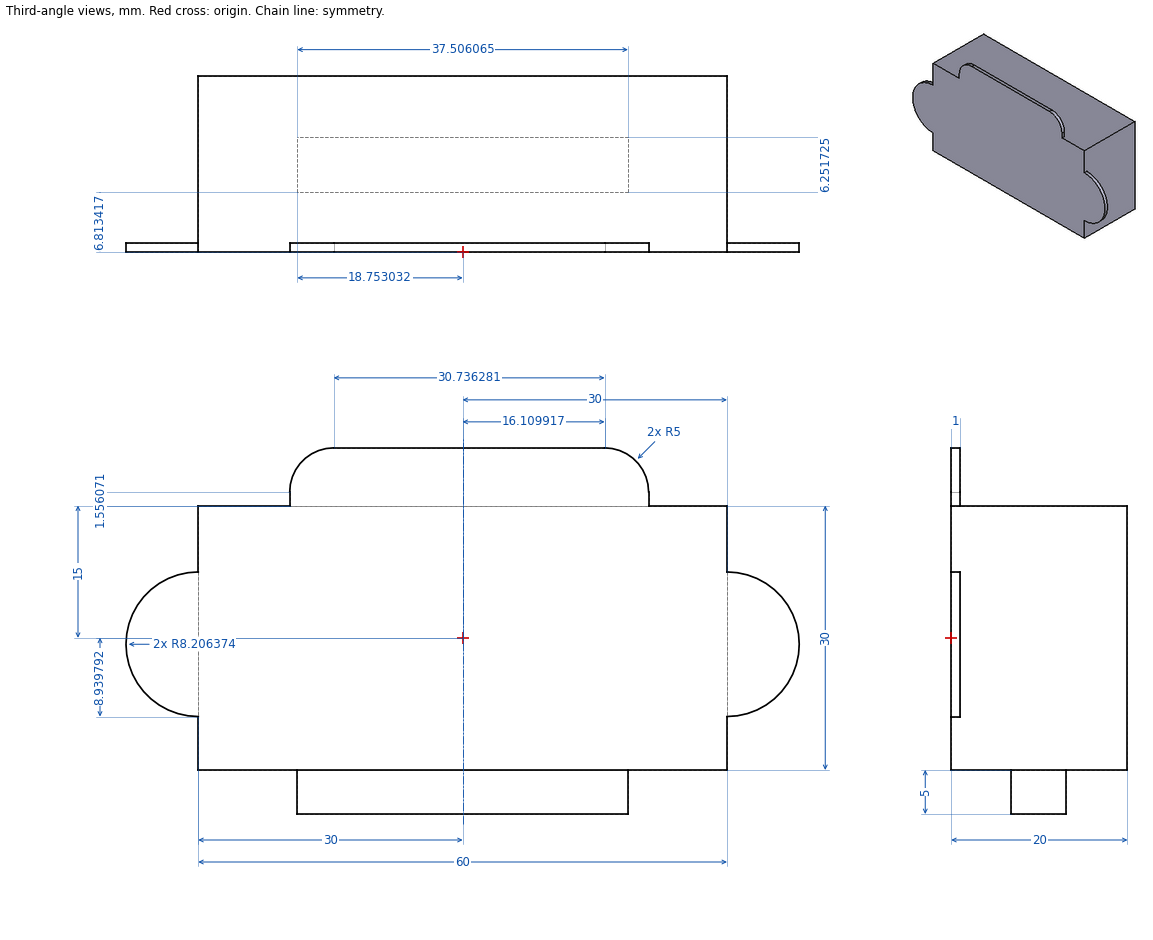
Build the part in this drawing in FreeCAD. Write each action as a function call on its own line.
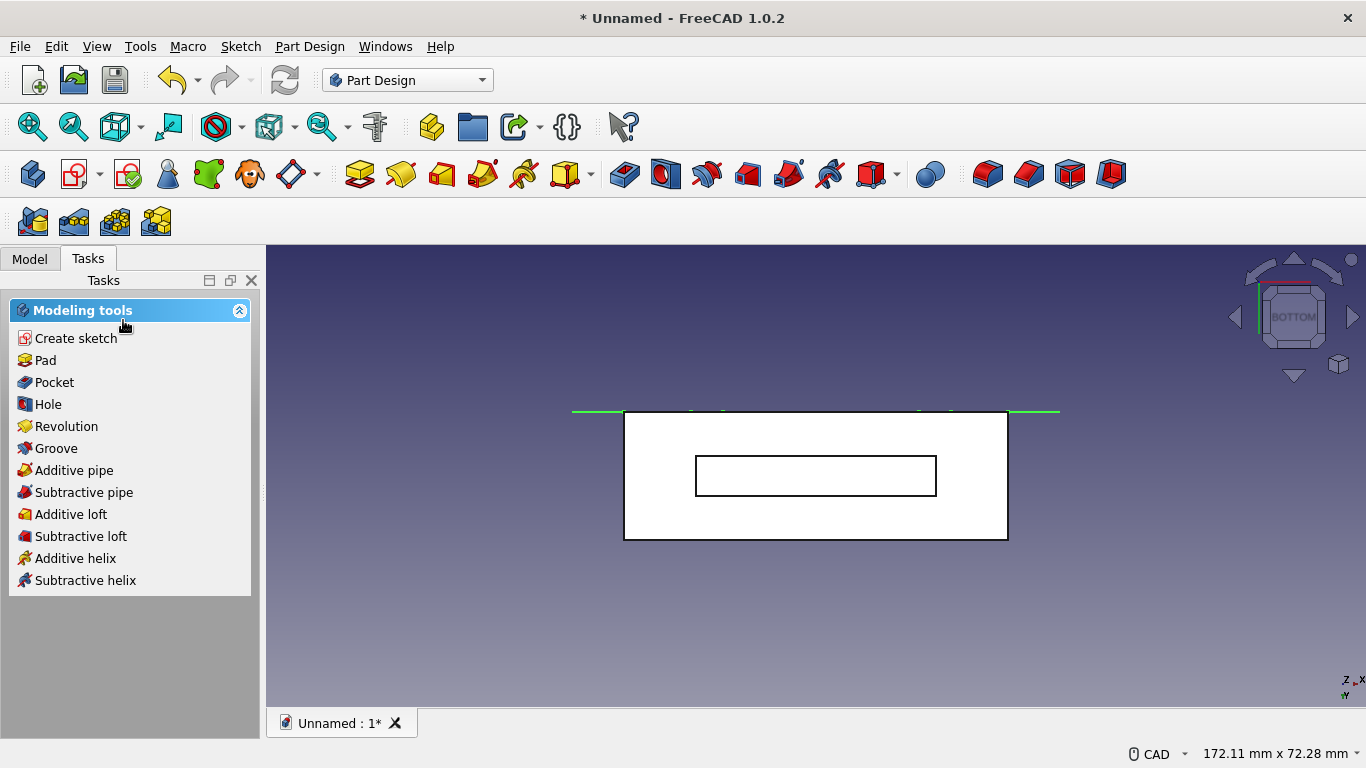
click(360, 174)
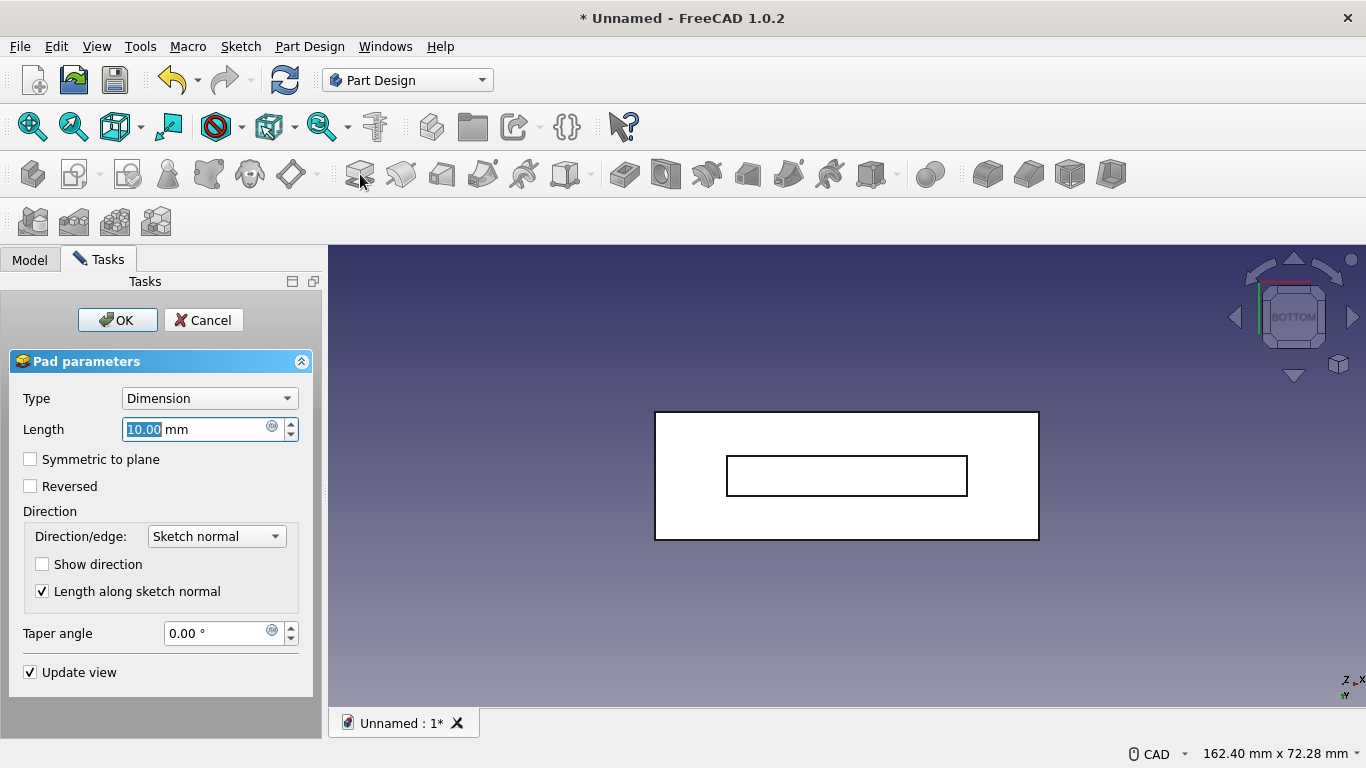
text(1)
key(Tab)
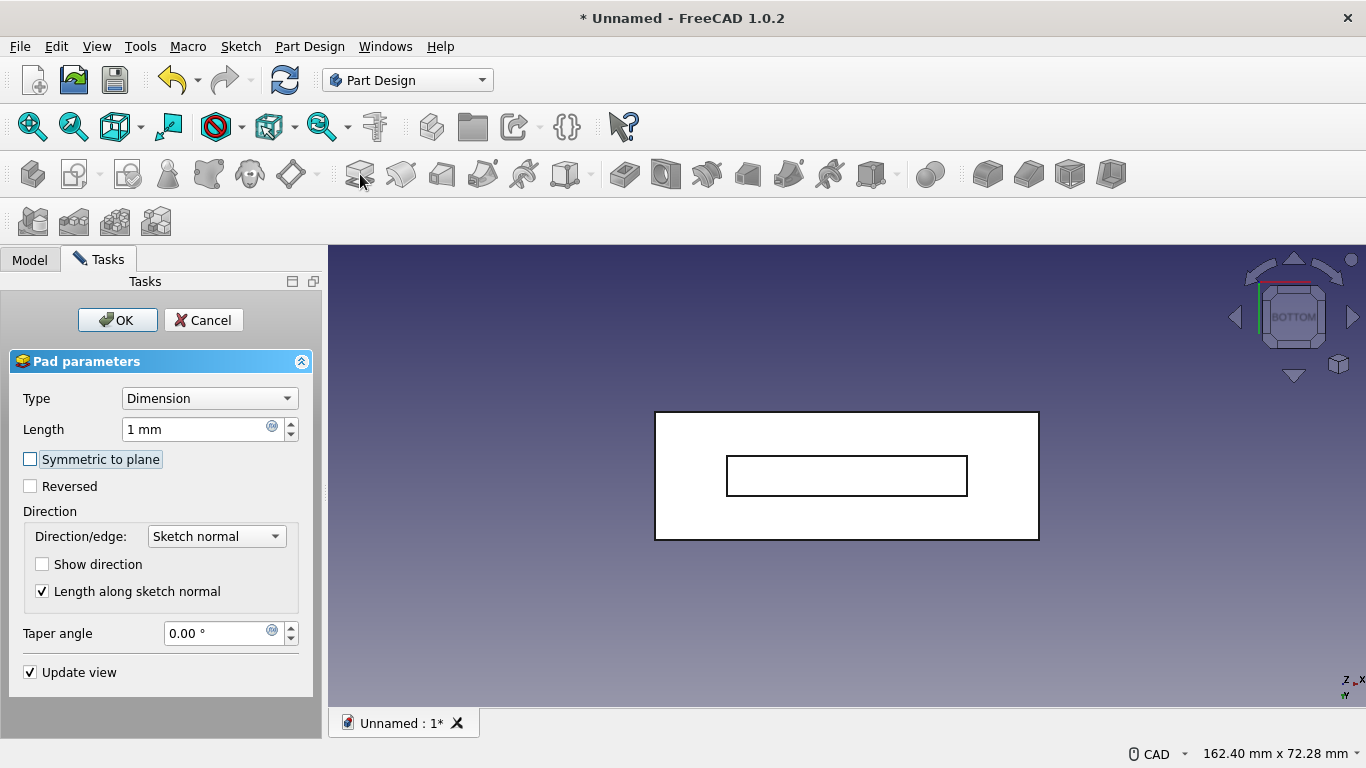
click(31, 486)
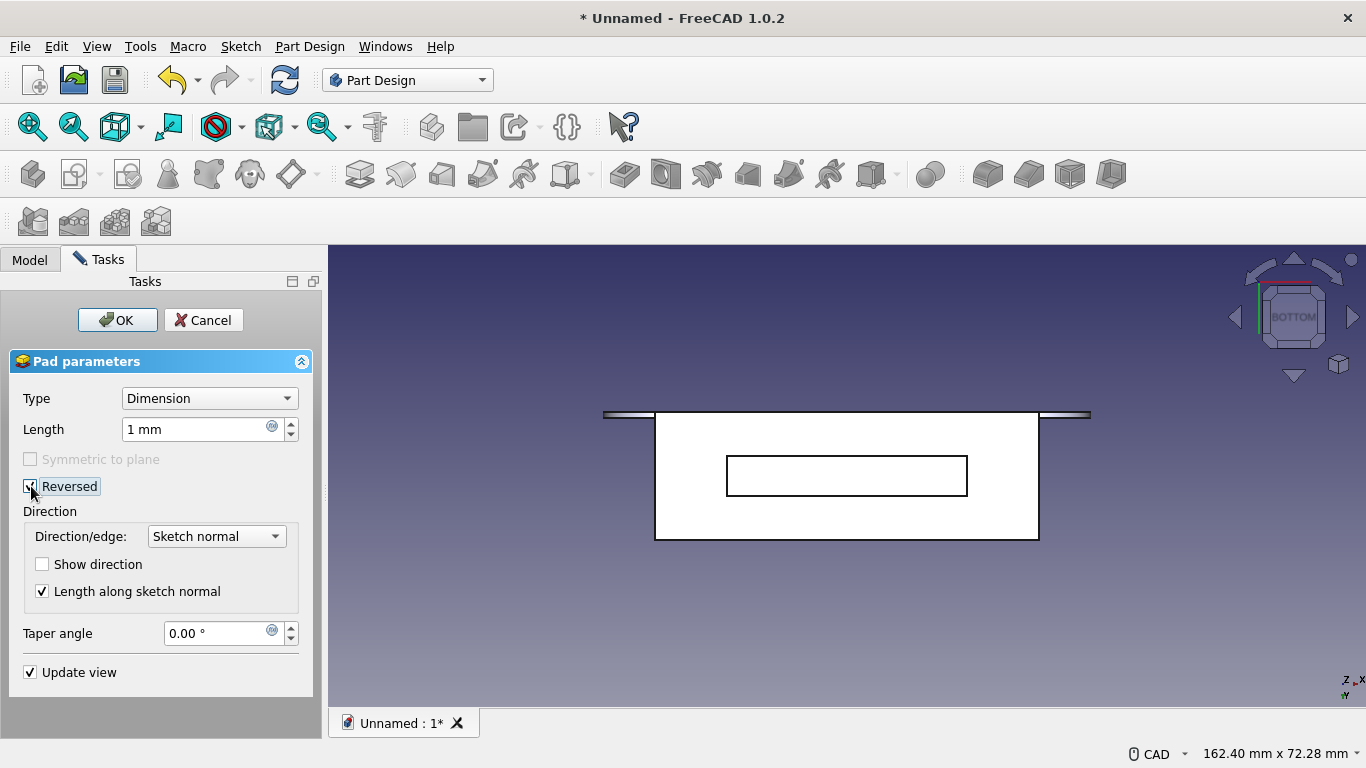
click(118, 320)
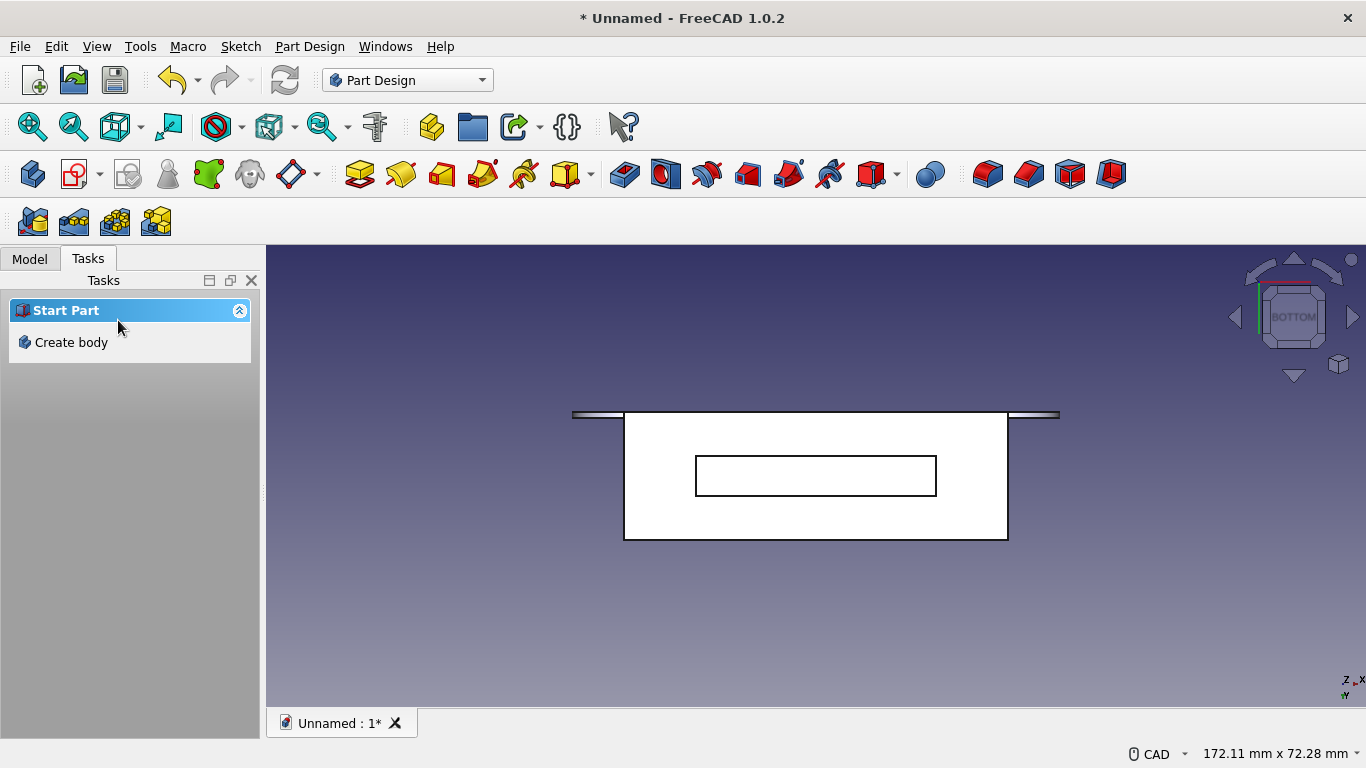
key(0)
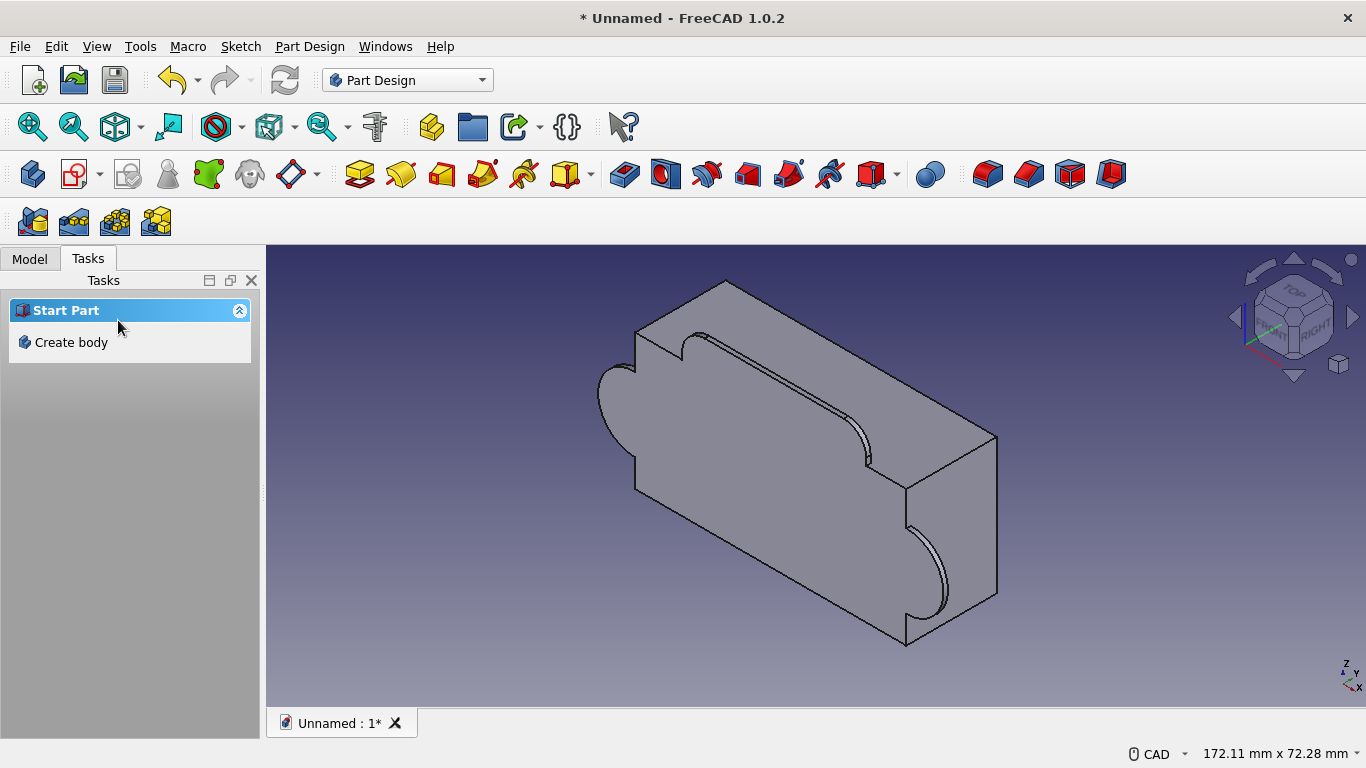
key(v)
key(f)